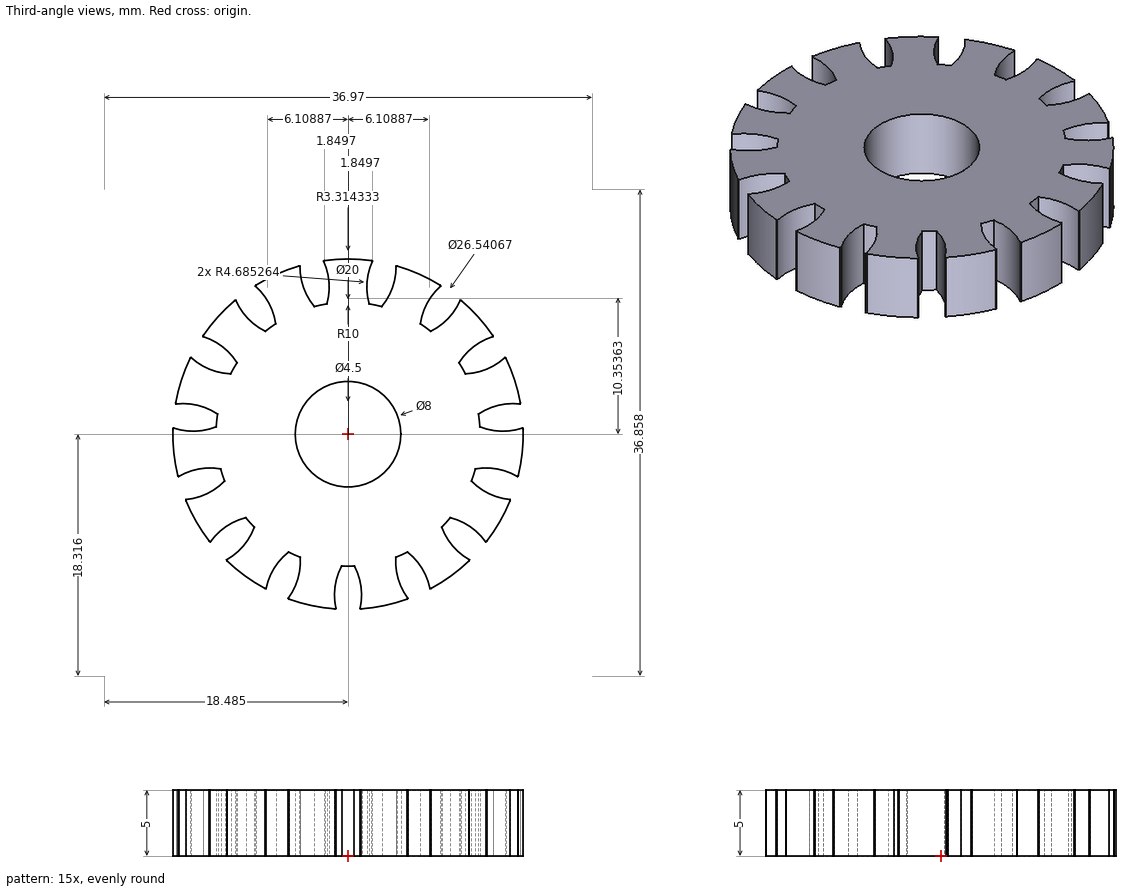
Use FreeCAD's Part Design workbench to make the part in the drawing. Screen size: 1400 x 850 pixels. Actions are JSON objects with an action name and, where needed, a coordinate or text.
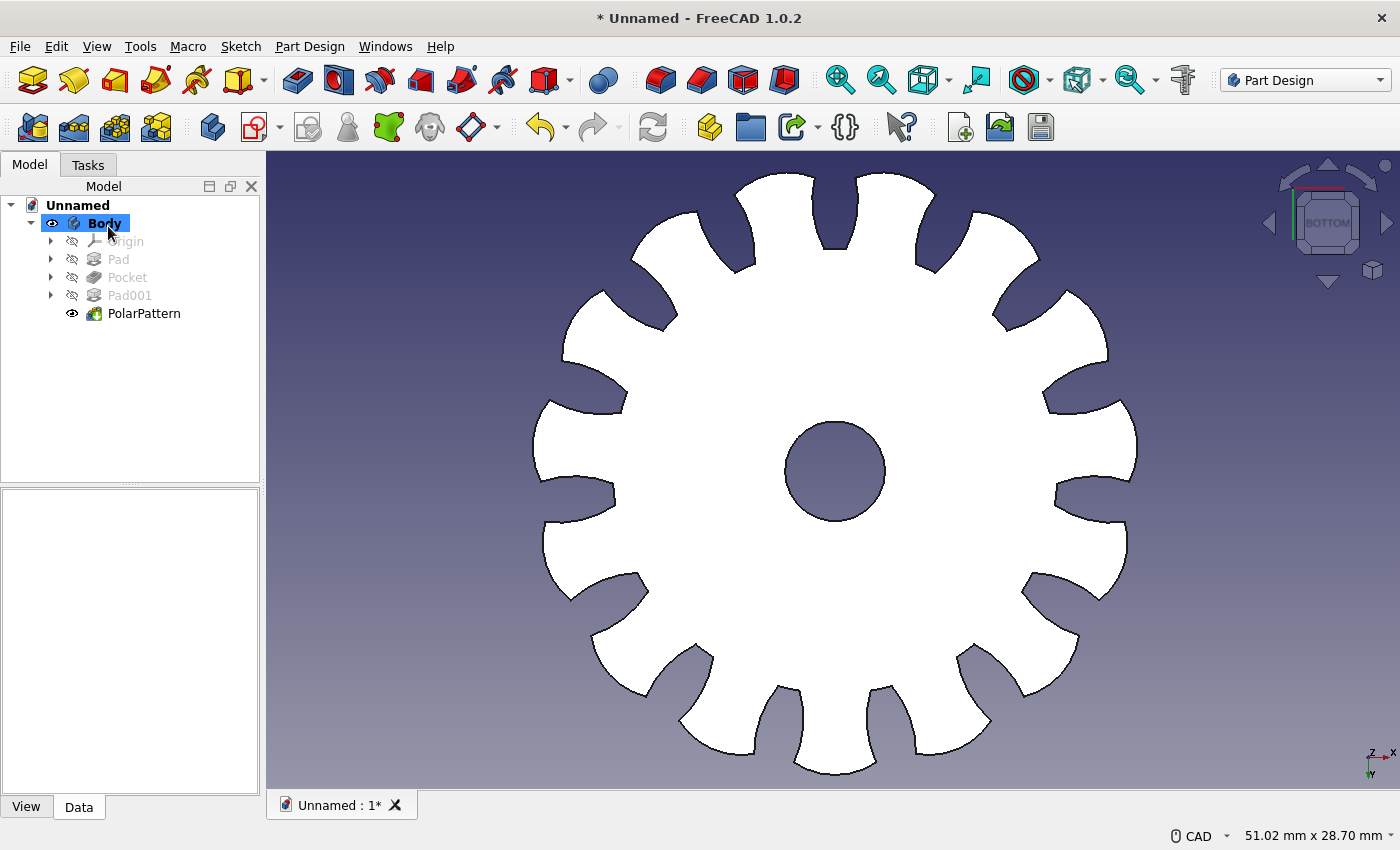
{"action": "left_click", "coordinate": [922, 559]}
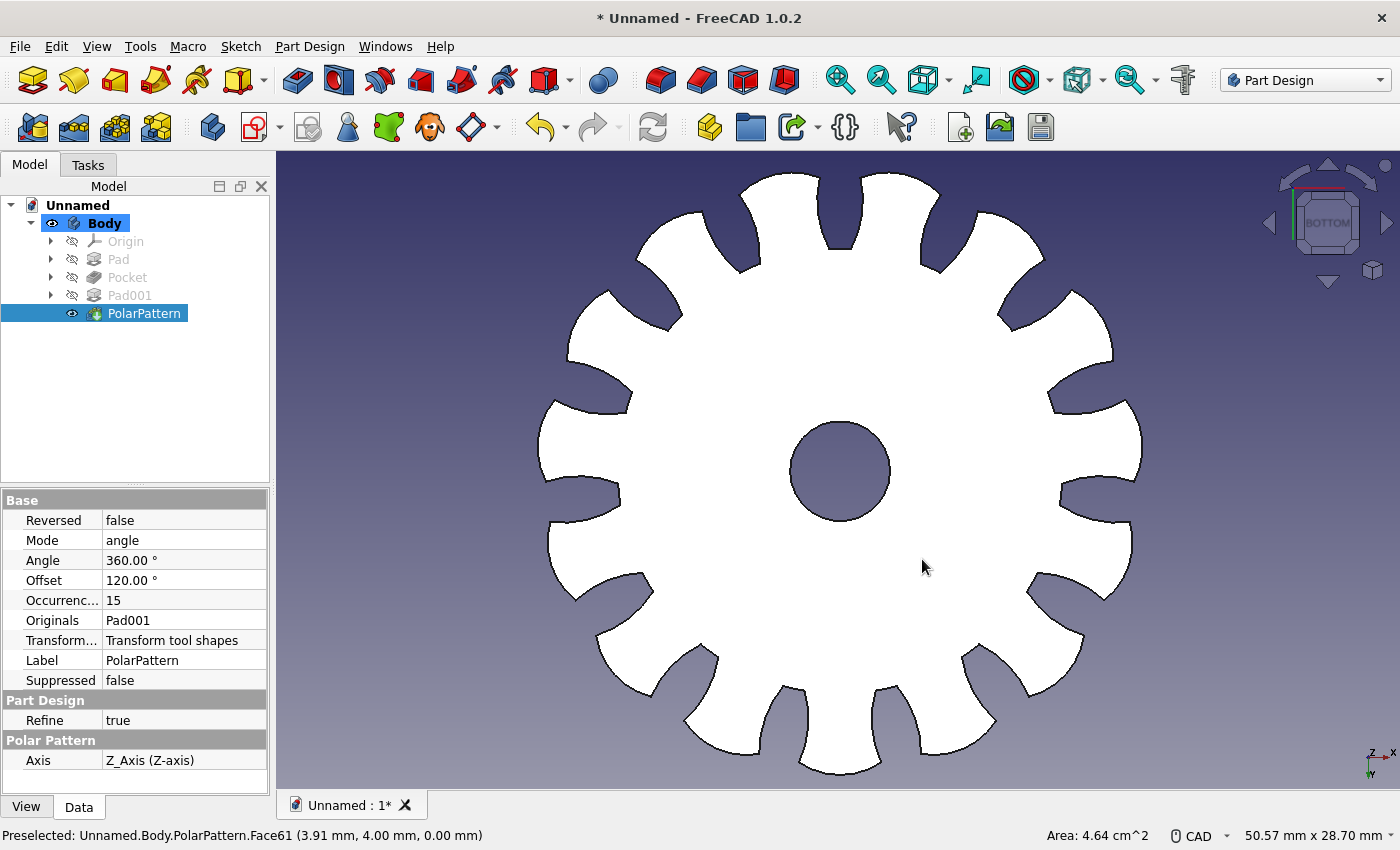
{"action": "left_click", "coordinate": [254, 128]}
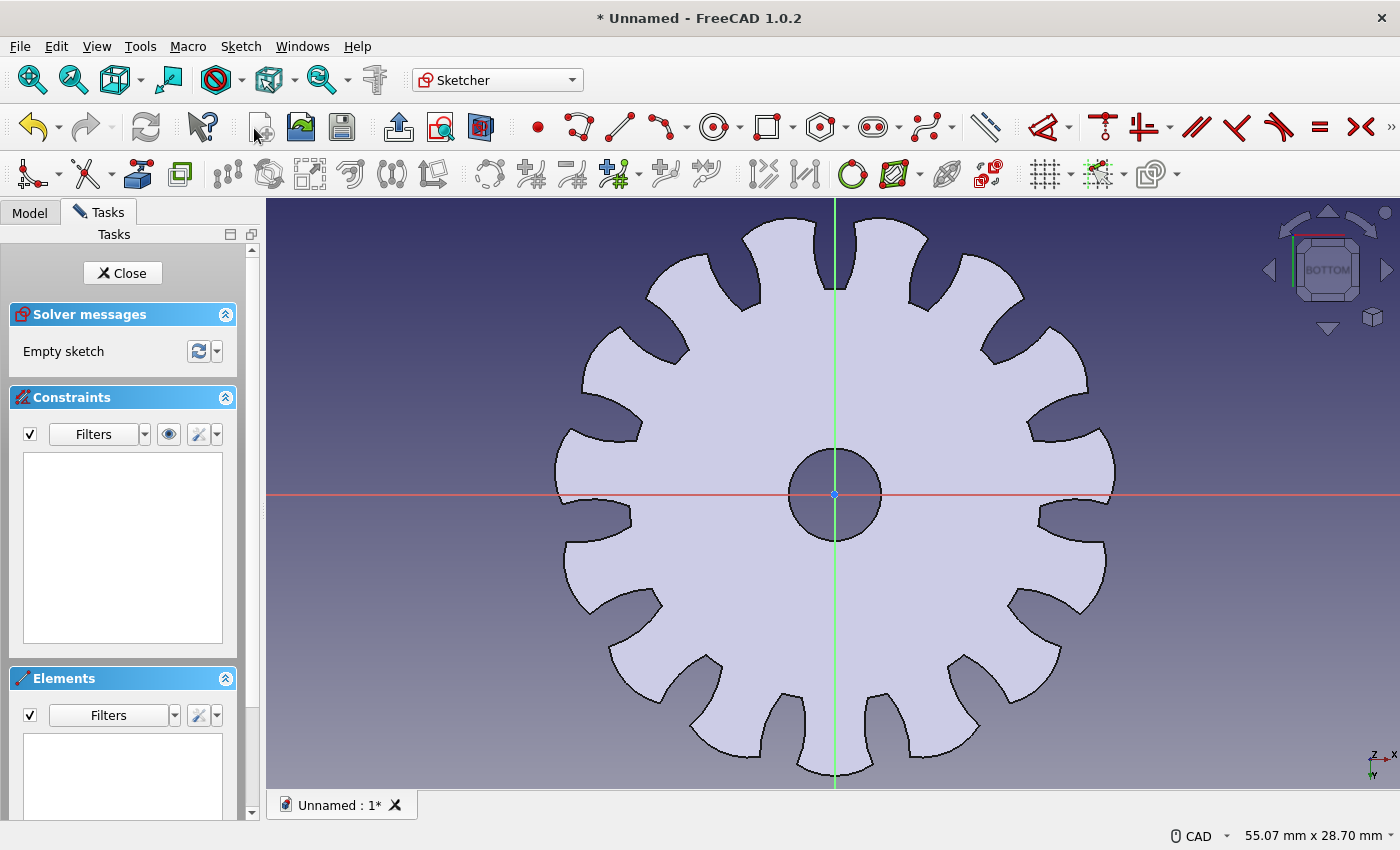
{"action": "scroll", "coordinate": [679, 489], "scroll_direction": "down", "scroll_amount": 3}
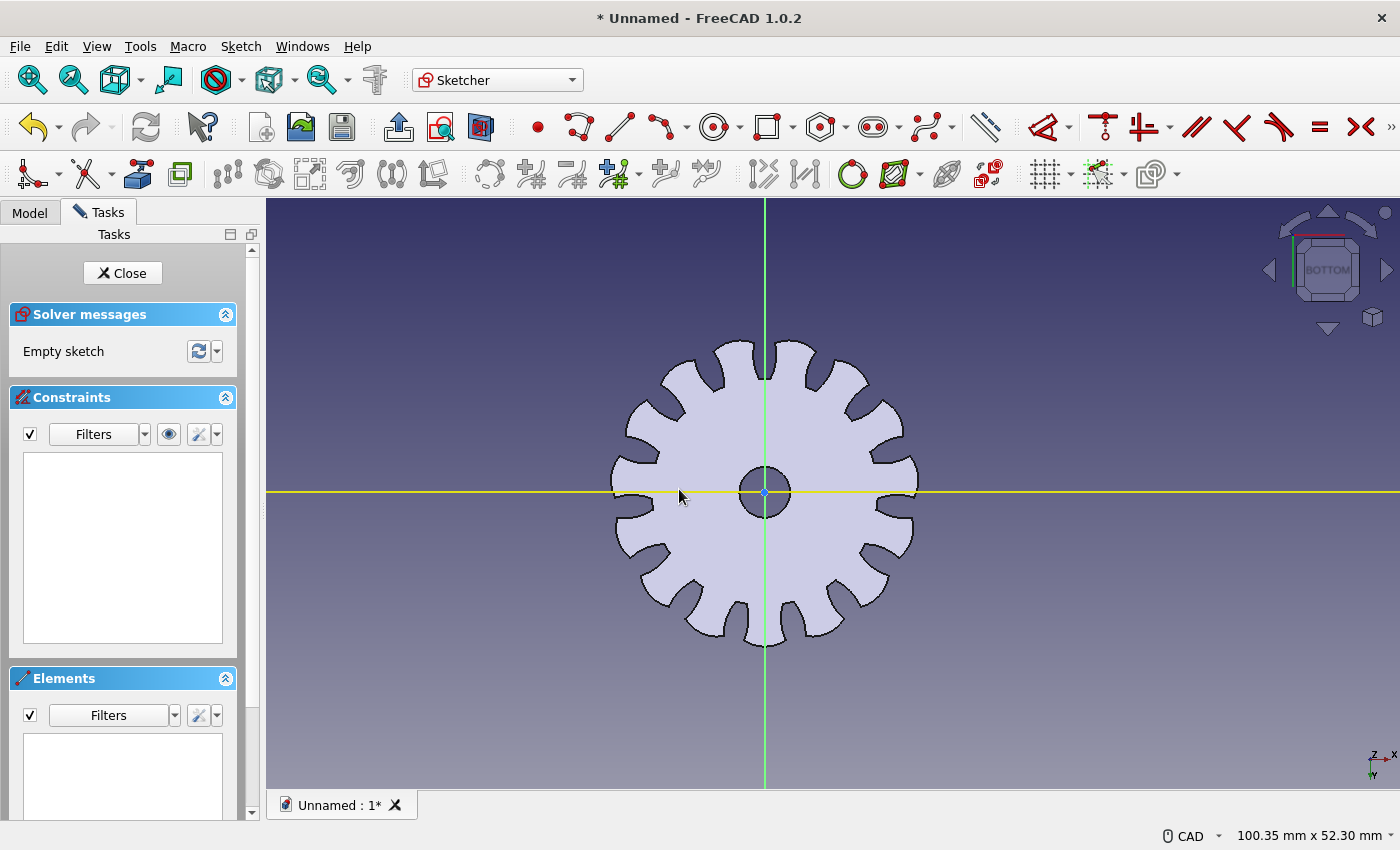
{"action": "key", "text": "g r"}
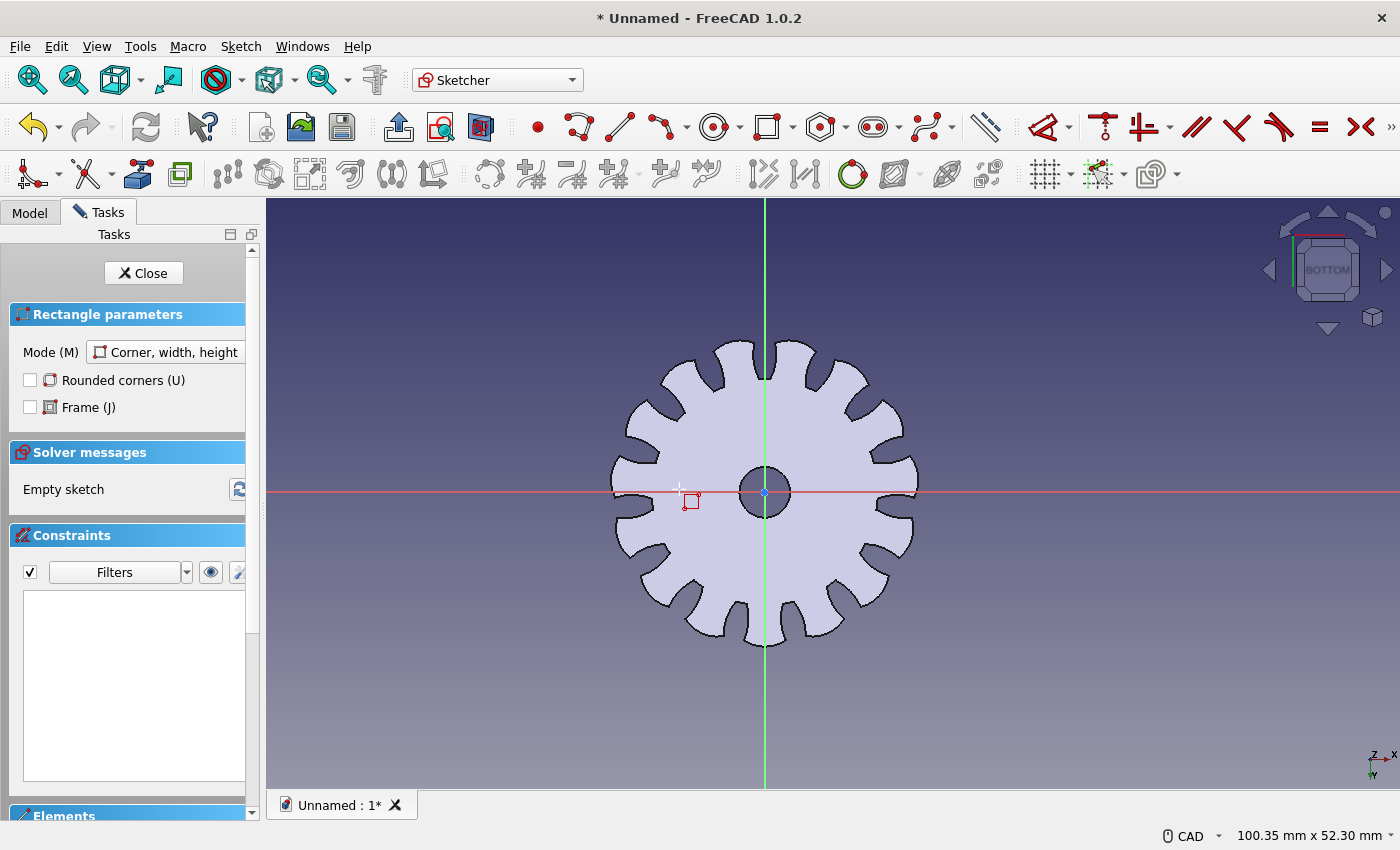
{"action": "left_click", "coordinate": [556, 285]}
{"action": "mouse_move", "coordinate": [974, 702]}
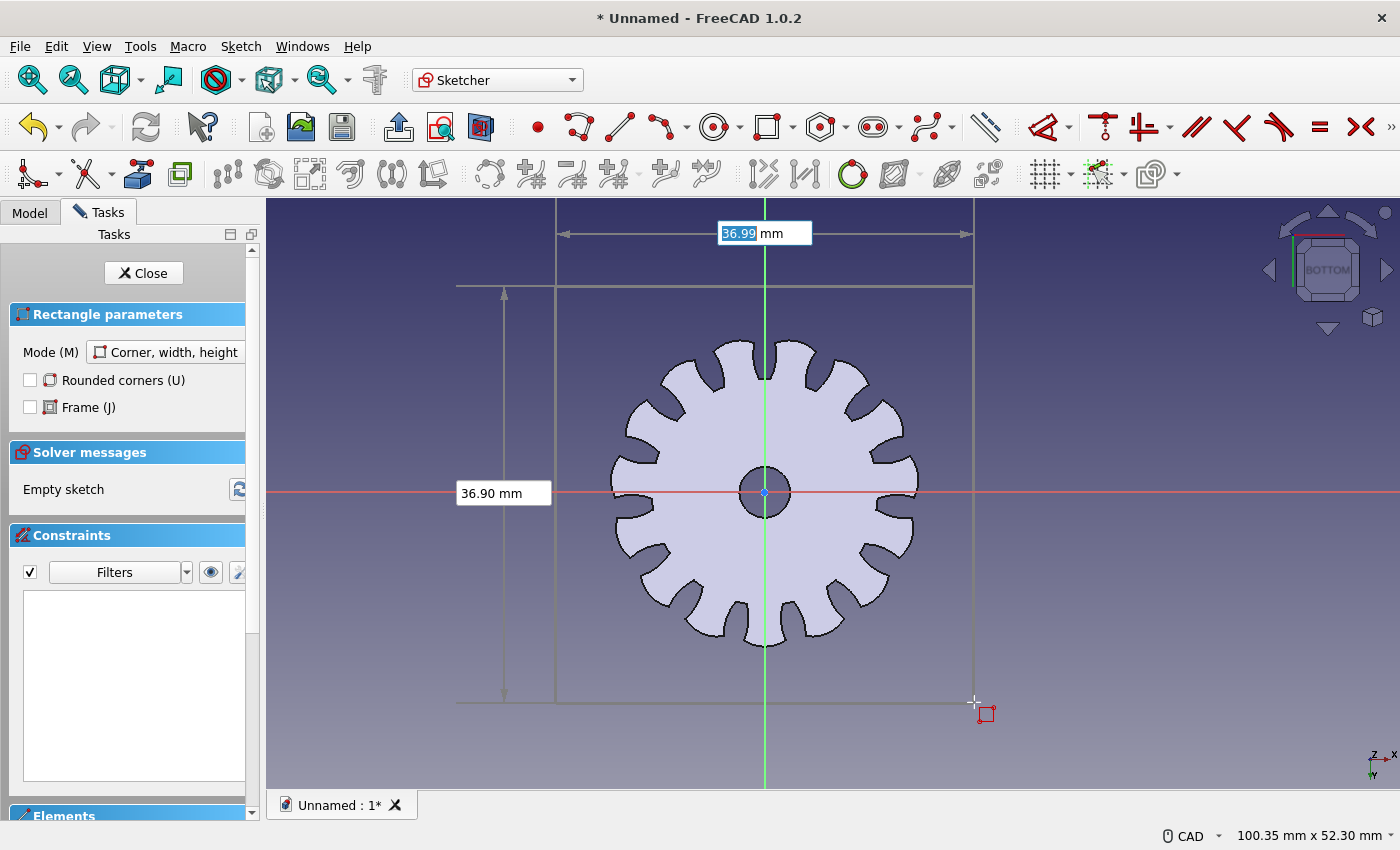
{"action": "type", "text": "36.97"}
{"action": "key", "text": "Tab"}
{"action": "type", "text": "36.858"}
{"action": "key", "text": "Return"}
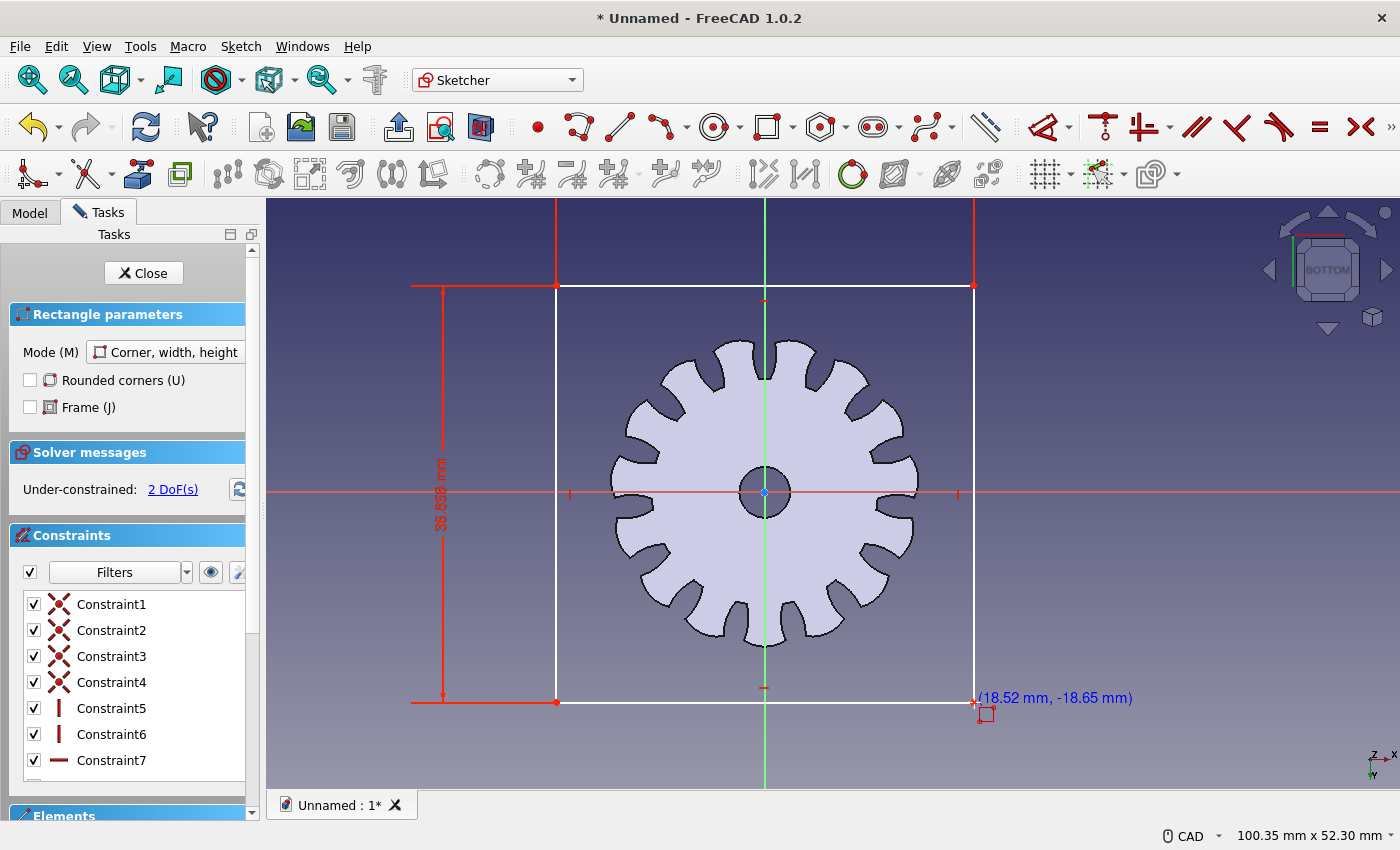
{"action": "key", "text": "g c"}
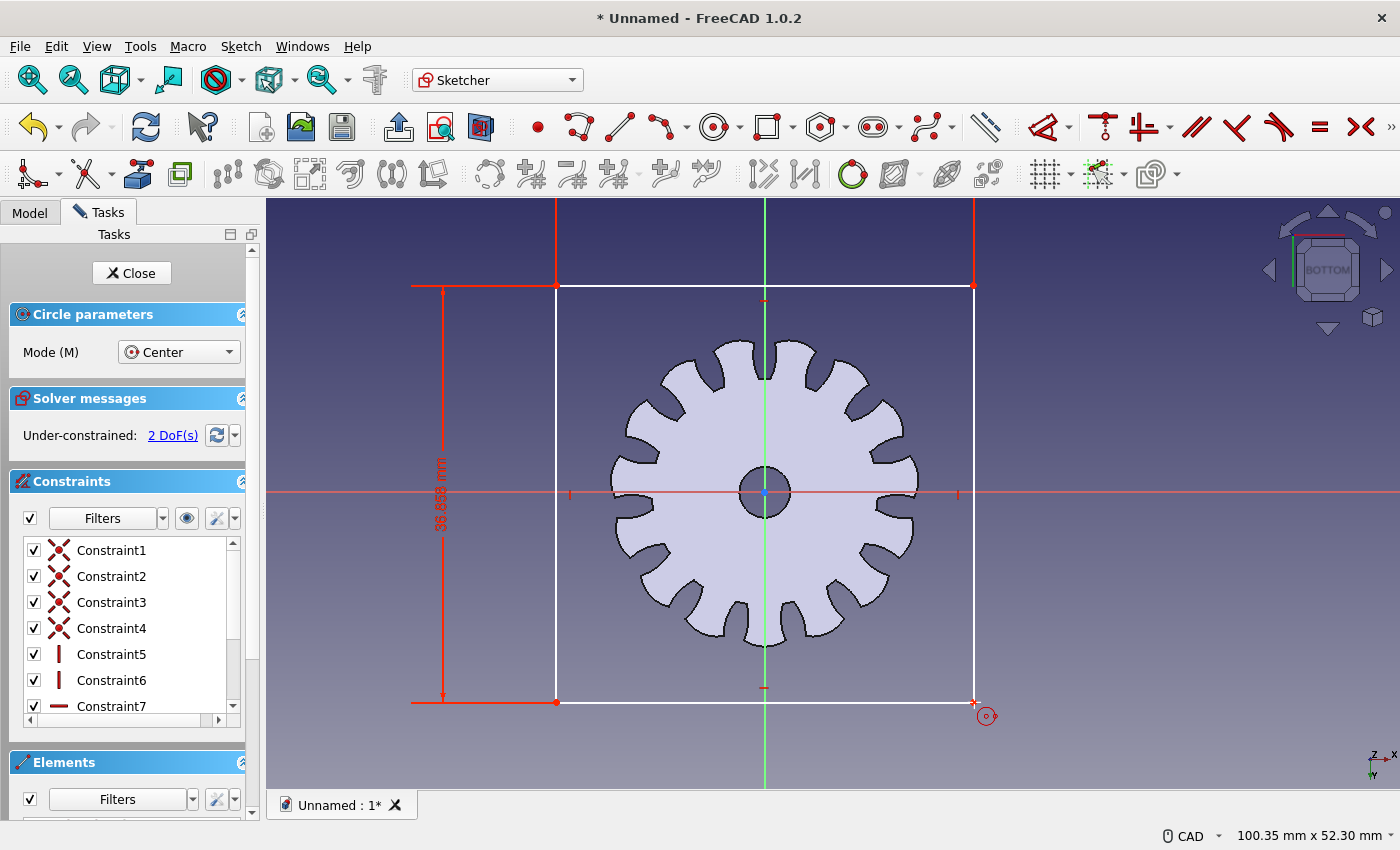
{"action": "left_click", "coordinate": [765, 492]}
{"action": "mouse_move", "coordinate": [871, 386]}